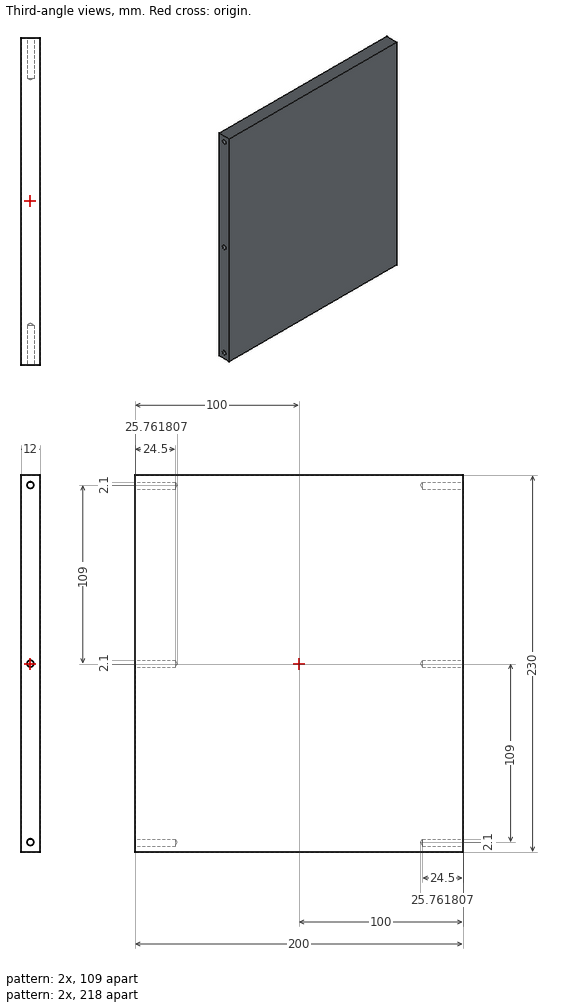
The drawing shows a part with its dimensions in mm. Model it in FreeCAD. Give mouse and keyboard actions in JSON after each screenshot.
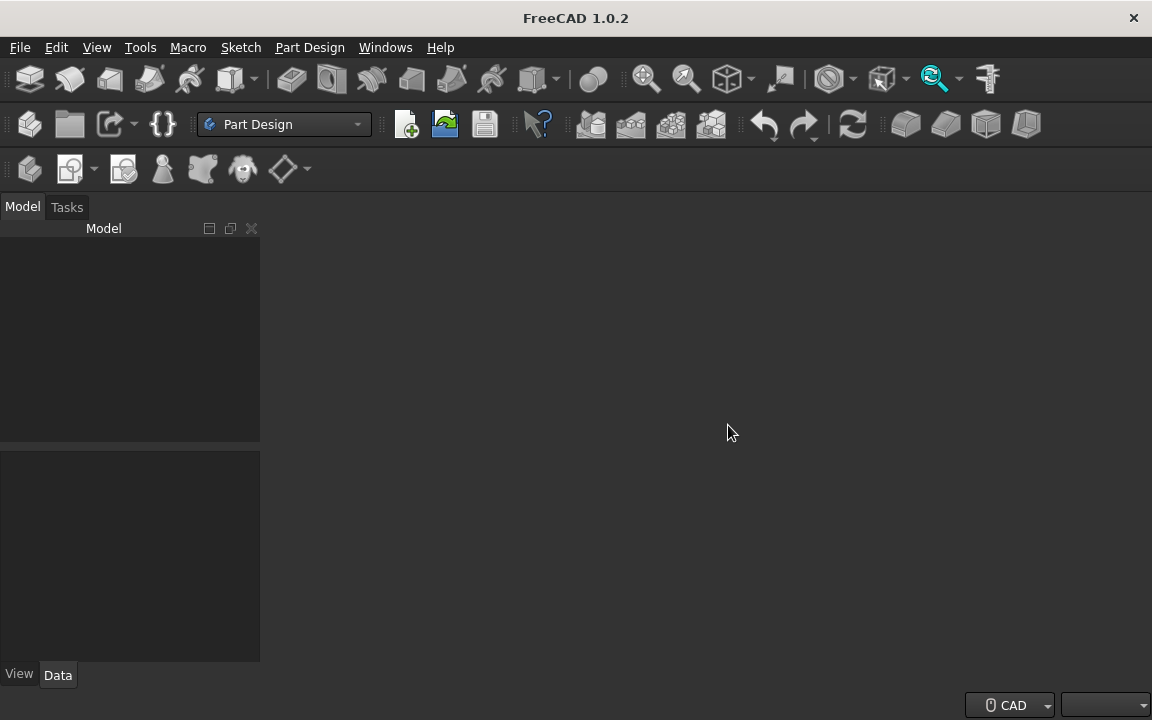
{"action": "left_click", "coordinate": [406, 124]}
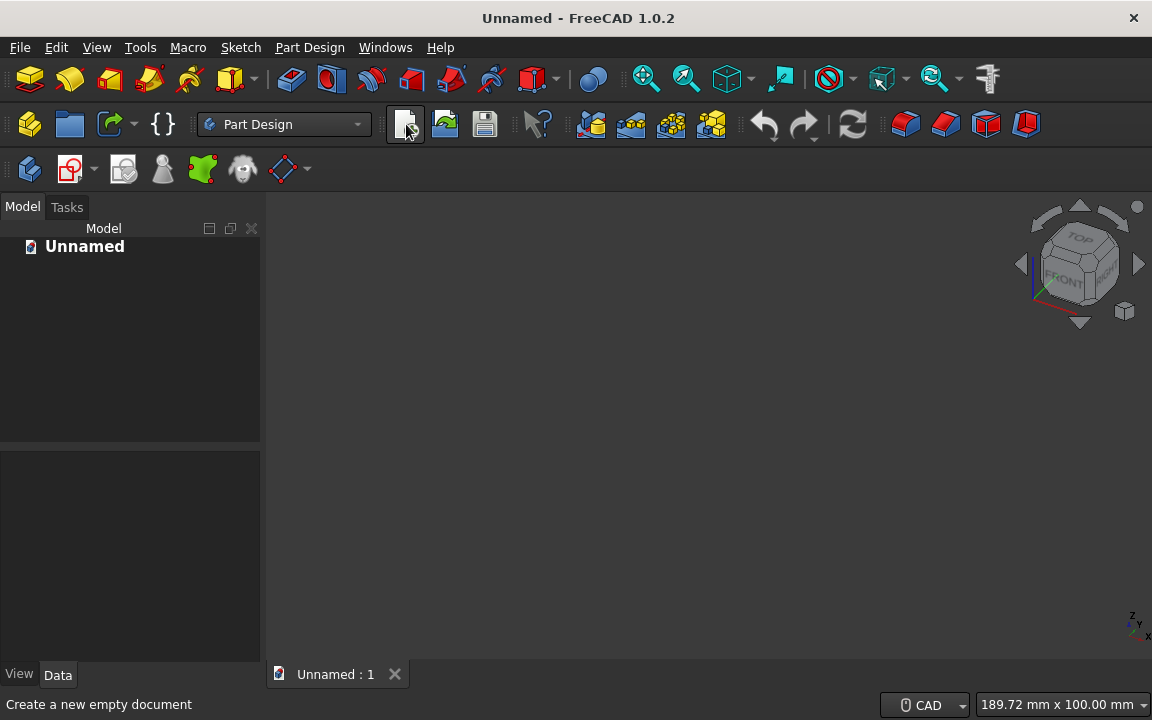
{"action": "left_click", "coordinate": [70, 170]}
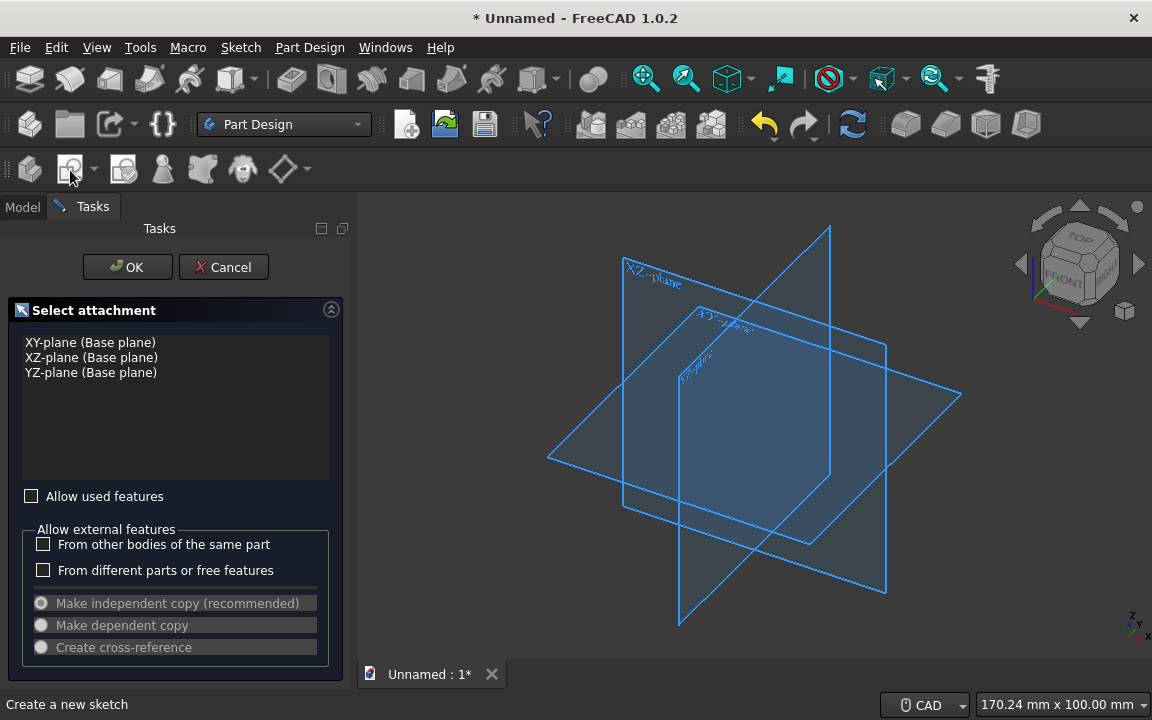
{"action": "left_click", "coordinate": [82, 372]}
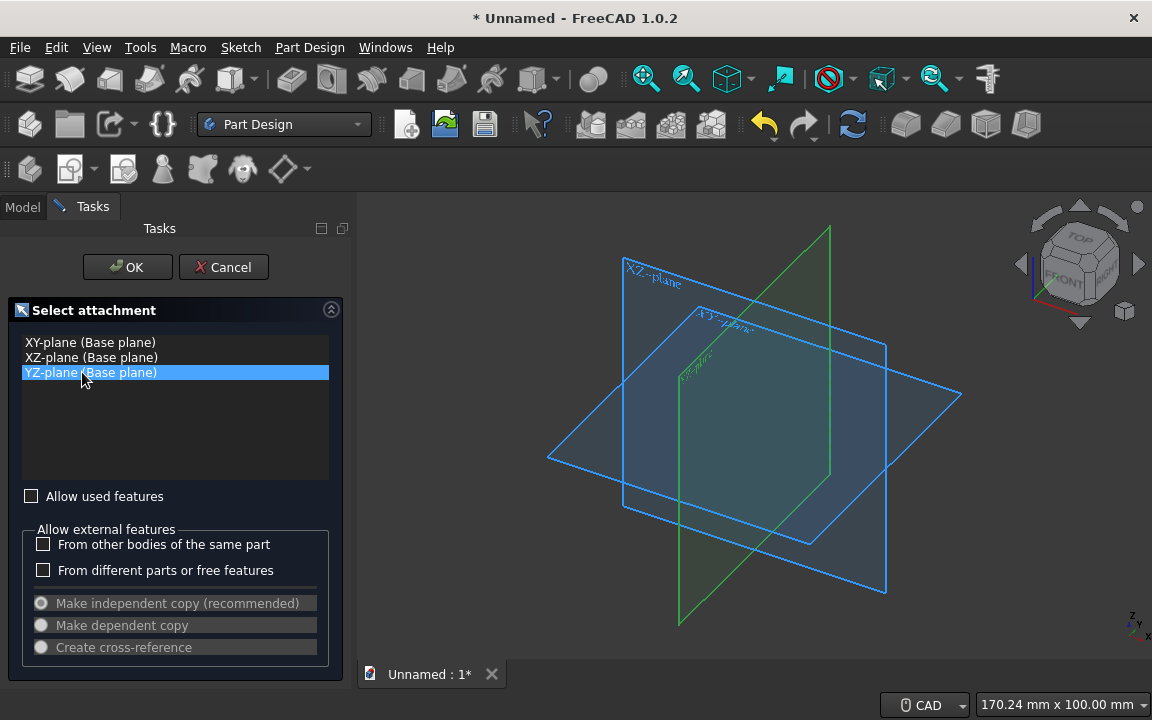
{"action": "left_click", "coordinate": [128, 267]}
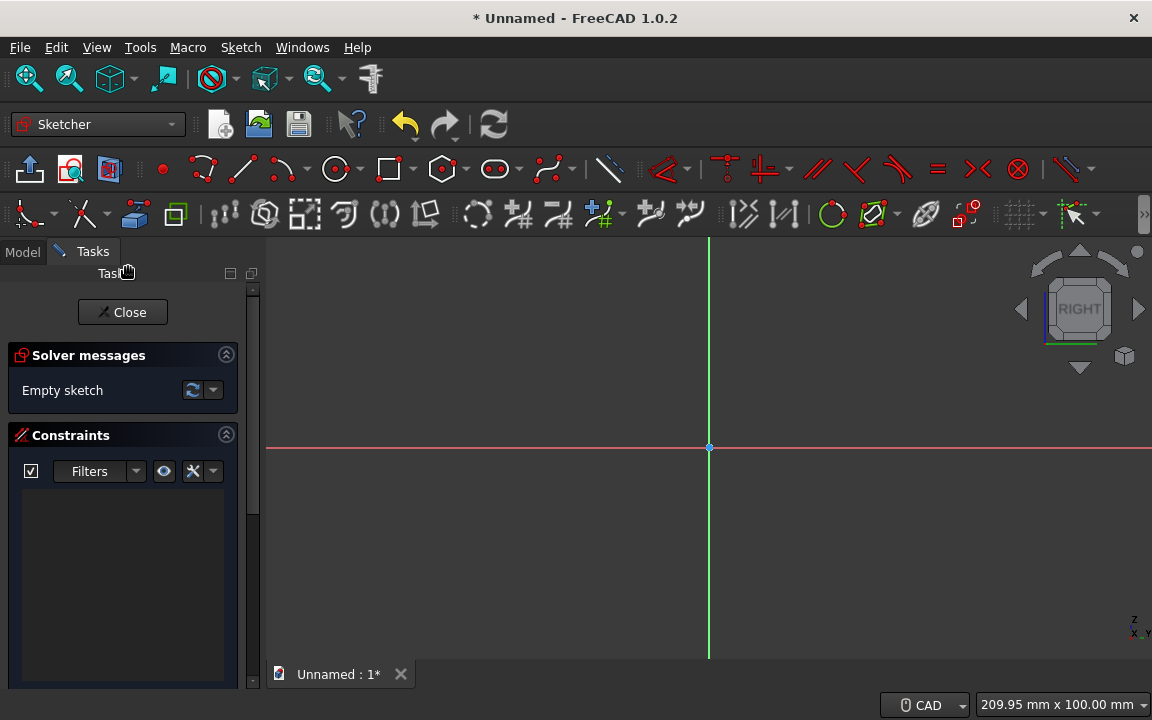
{"action": "scroll", "coordinate": [618, 448], "scroll_direction": "down", "scroll_amount": 7}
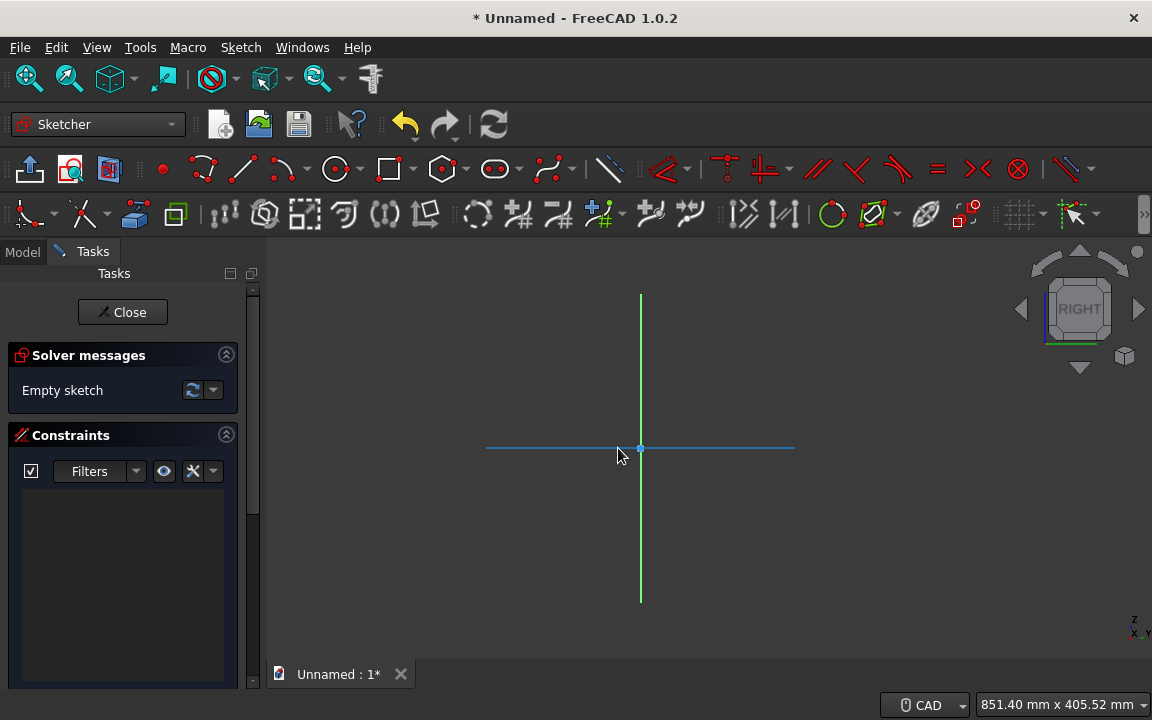
{"action": "left_click", "coordinate": [416, 170]}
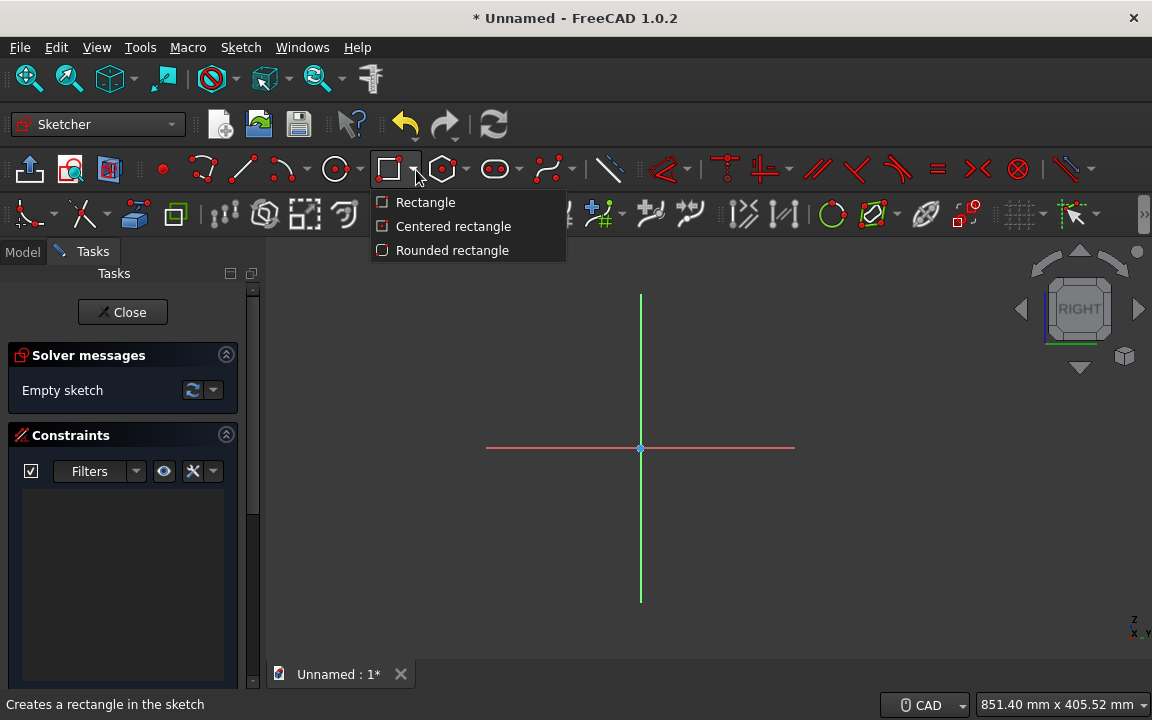
{"action": "left_click", "coordinate": [468, 226]}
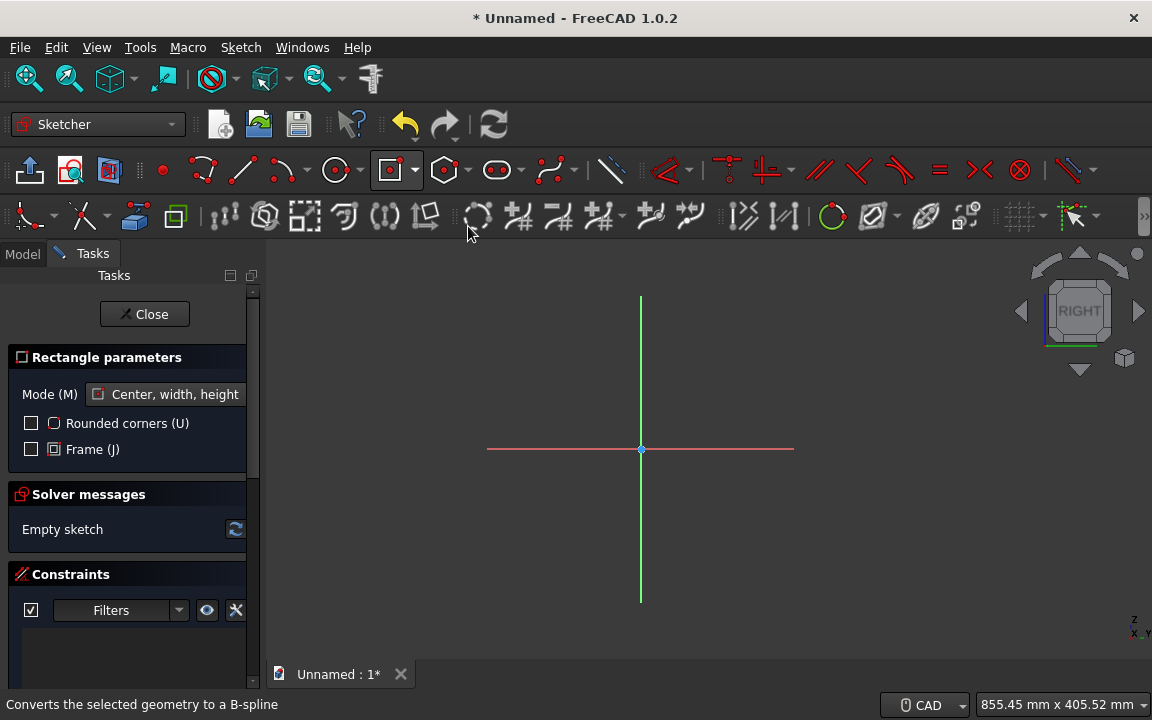
{"action": "left_click", "coordinate": [641, 449]}
{"action": "mouse_move", "coordinate": [745, 330]}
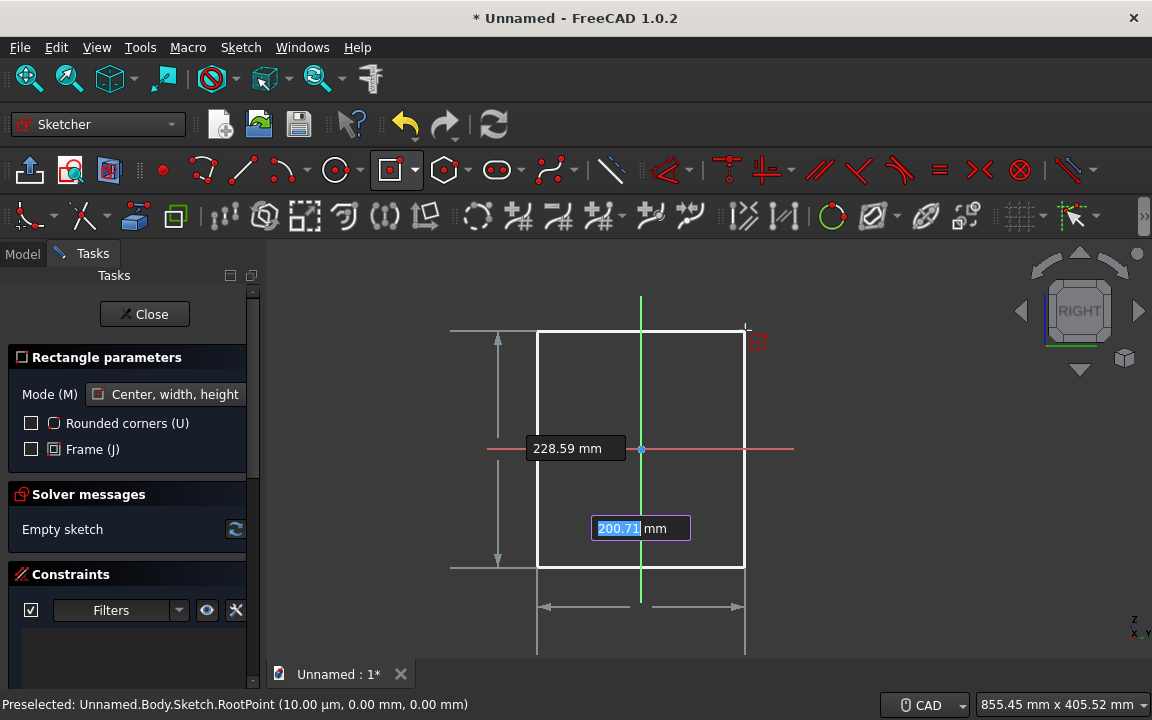
{"action": "type", "text": "200"}
{"action": "key", "text": "Tab"}
{"action": "type", "text": "230"}
{"action": "key", "text": "Return"}
{"action": "key", "text": "Escape"}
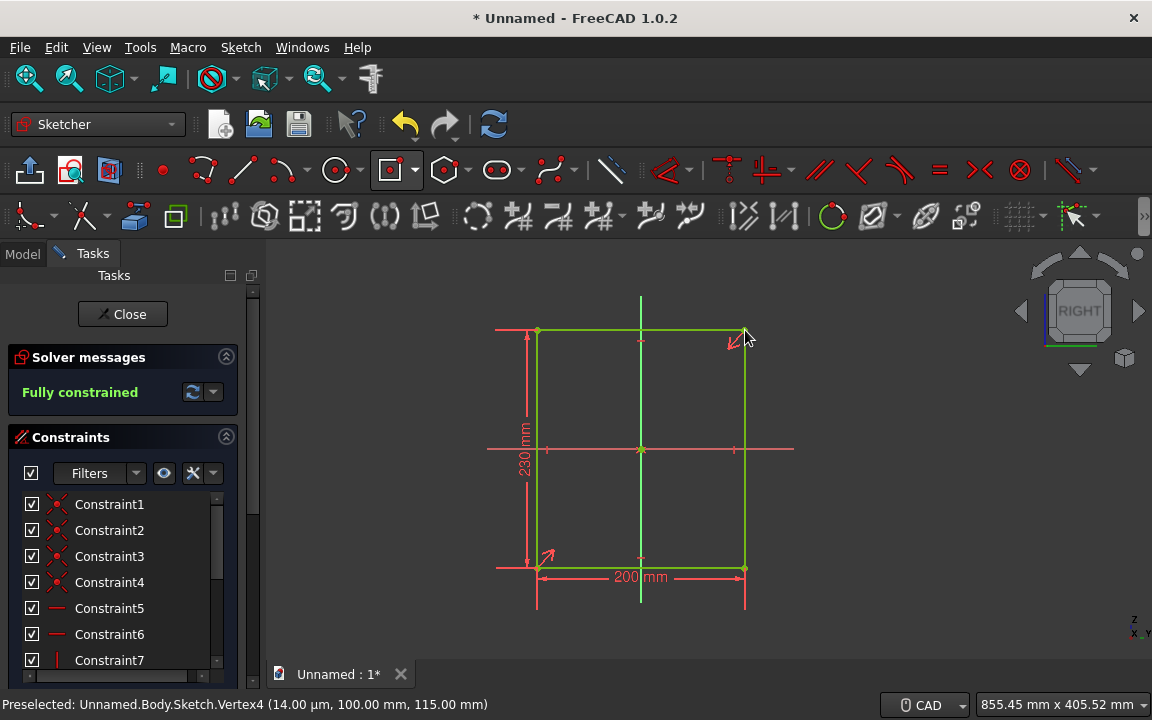
{"action": "left_click", "coordinate": [123, 314]}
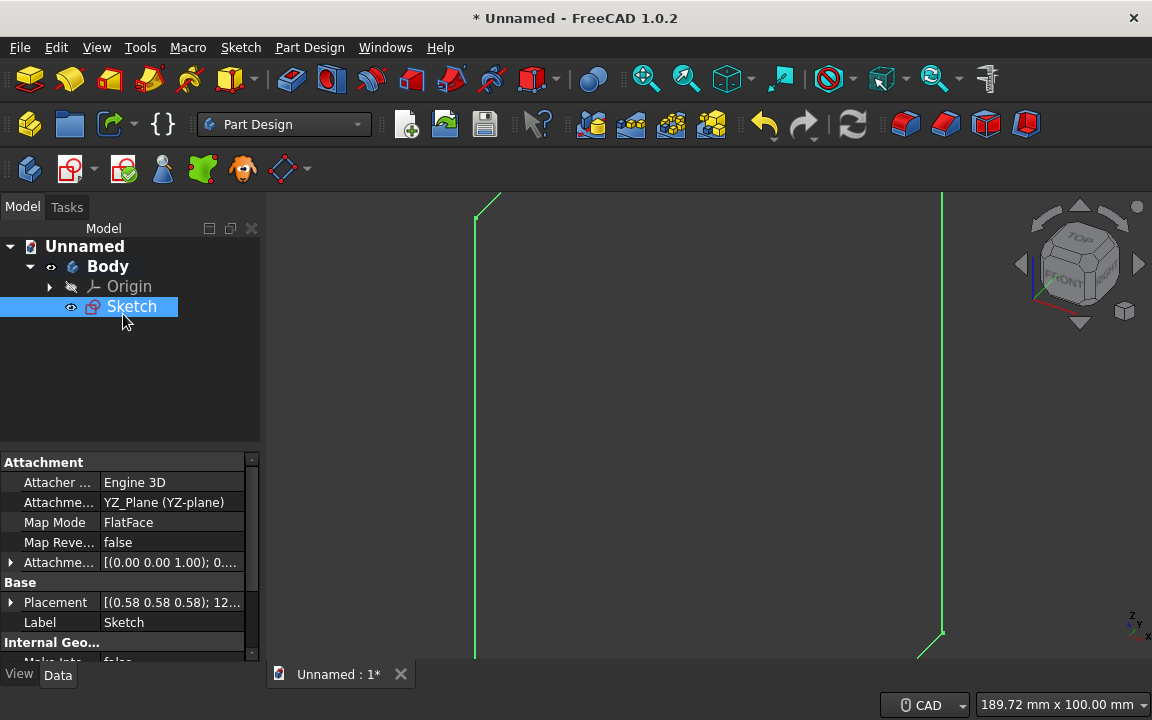
{"action": "left_click", "coordinate": [30, 80]}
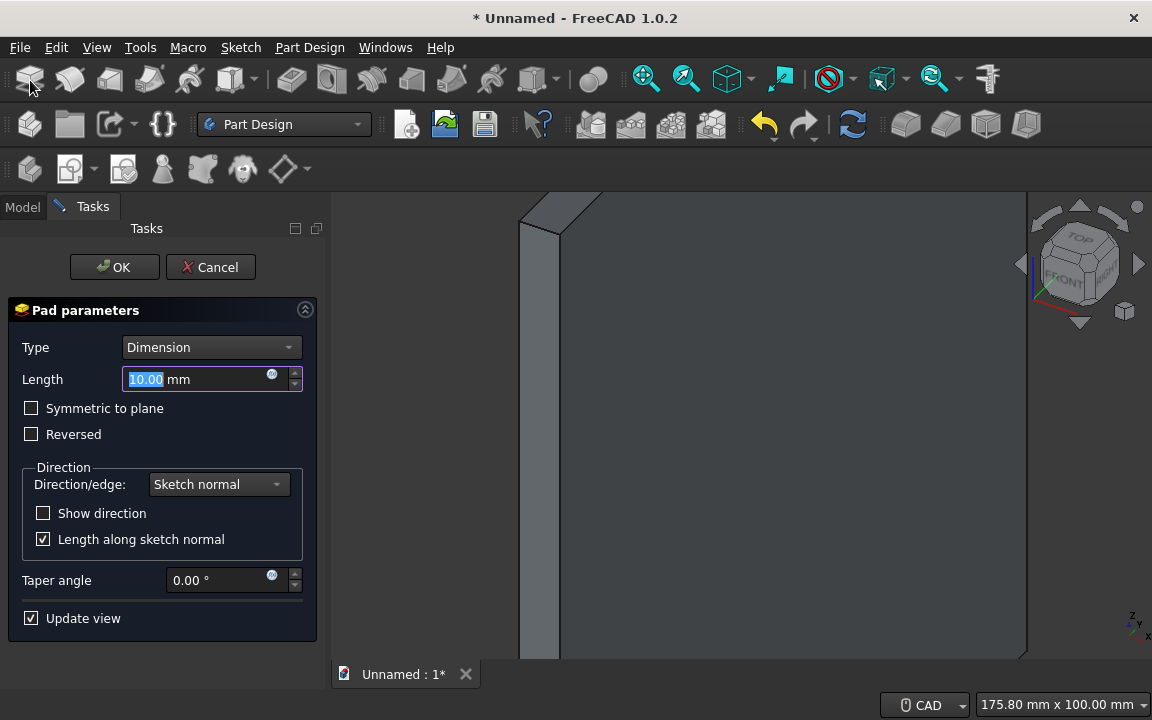
{"action": "type", "text": "12"}
{"action": "key", "text": "Tab"}